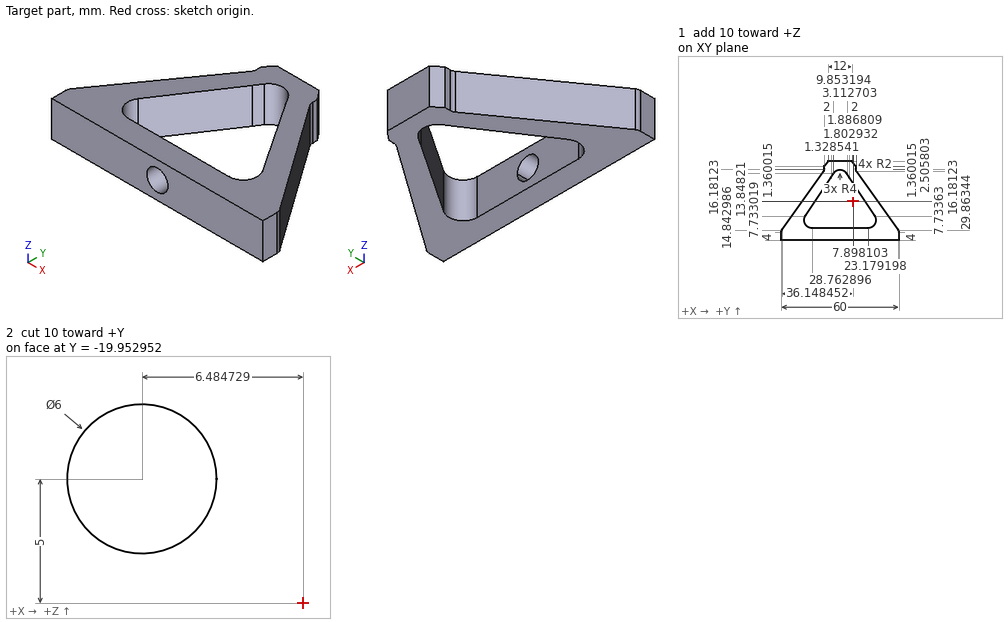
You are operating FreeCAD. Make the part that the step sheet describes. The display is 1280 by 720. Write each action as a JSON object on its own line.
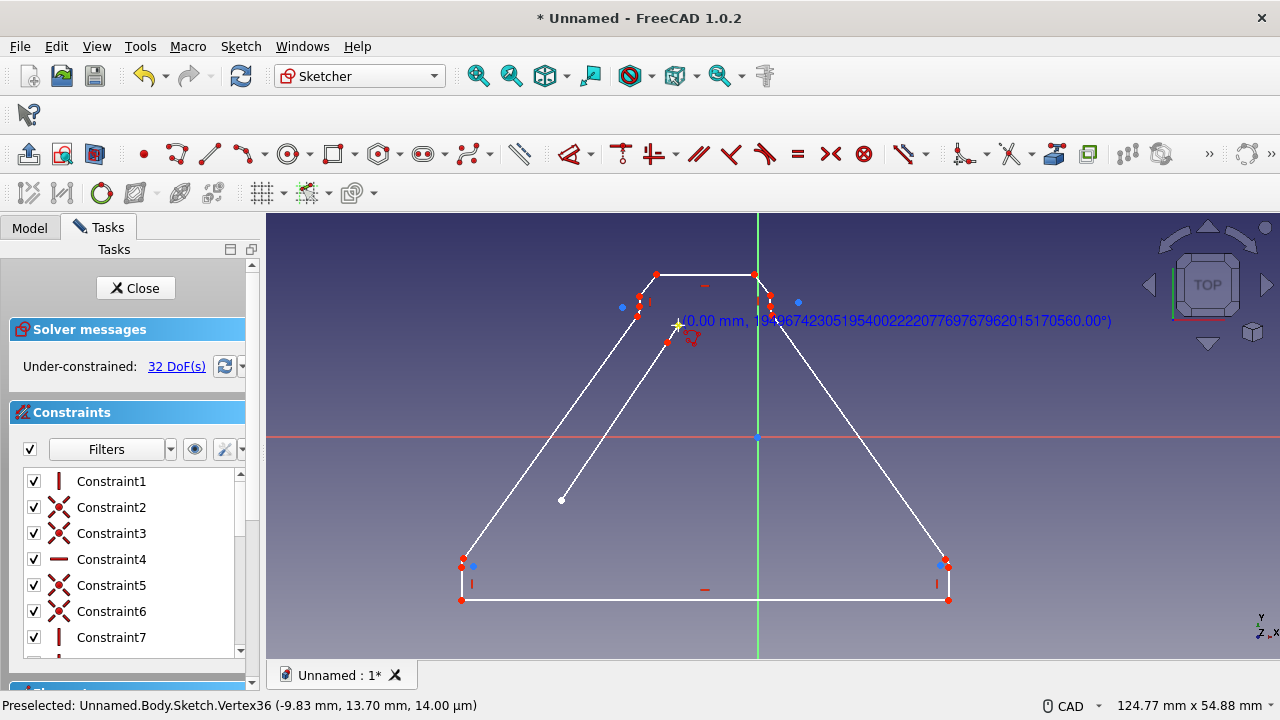
{"action": "left_click", "coordinate": [733, 325]}
{"action": "left_click", "coordinate": [743, 341]}
{"action": "left_click", "coordinate": [849, 500]}
{"action": "right_click", "coordinate": [849, 500]}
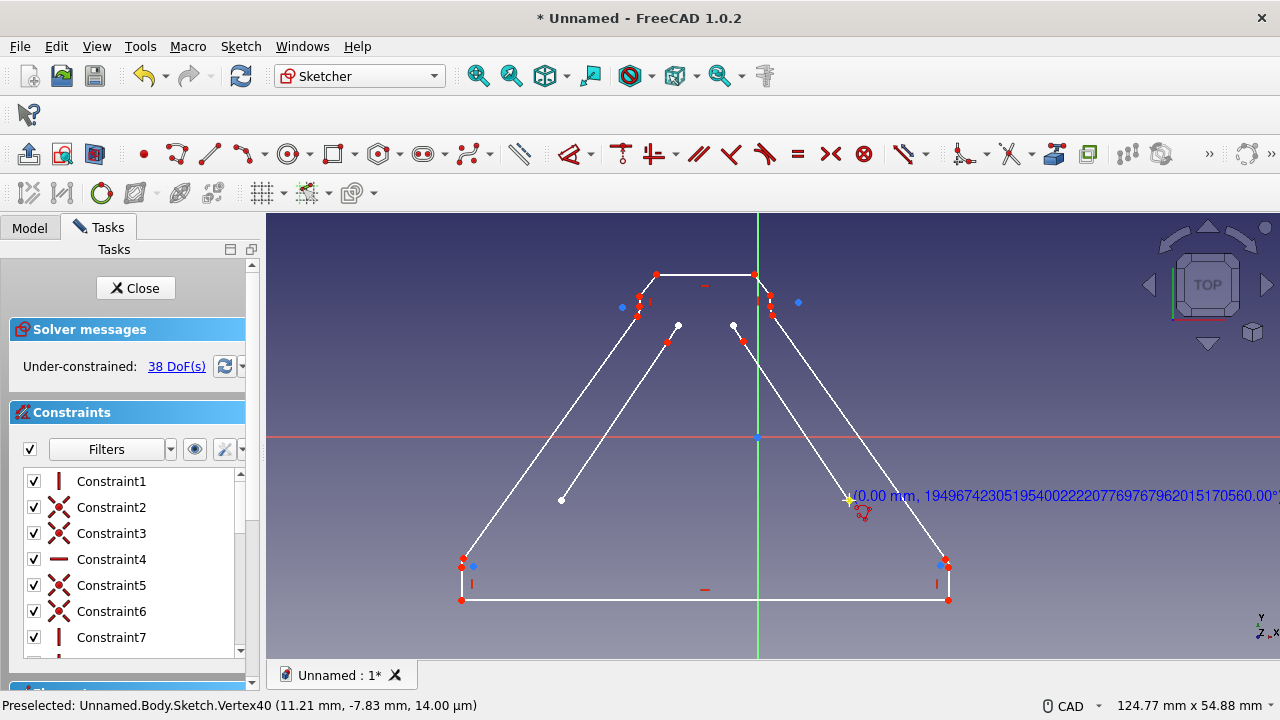
{"action": "left_click", "coordinate": [210, 154]}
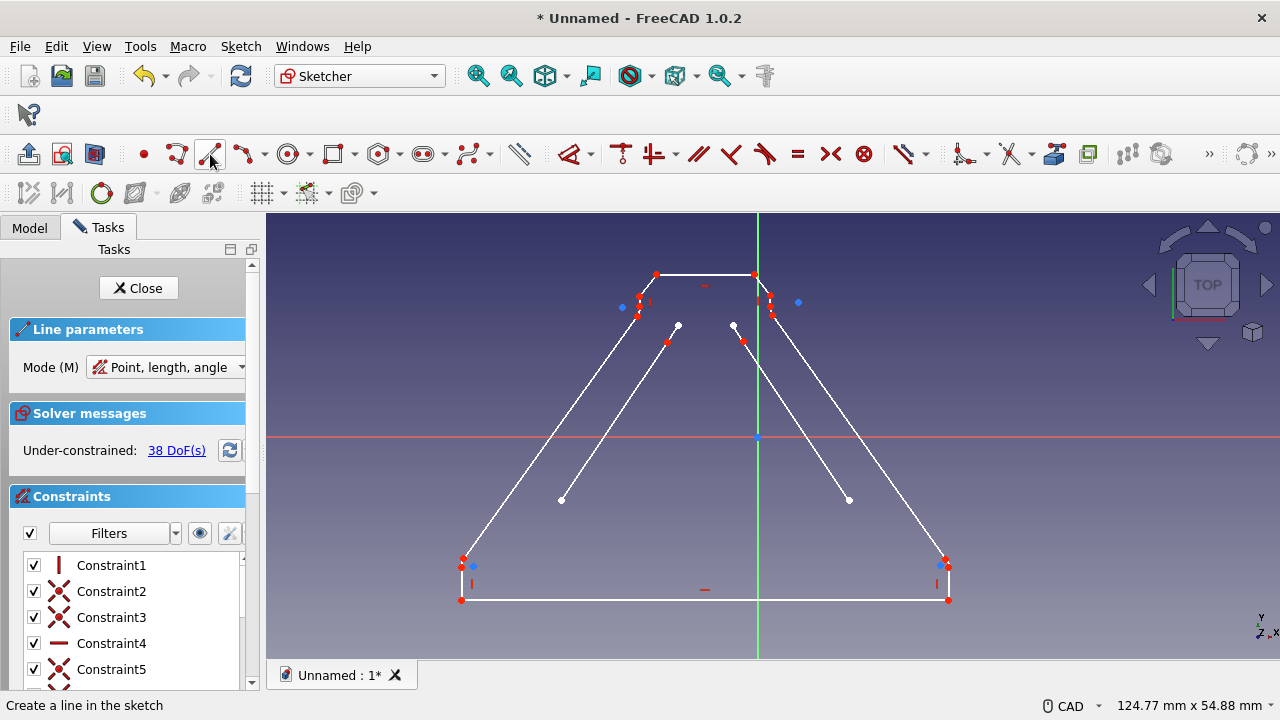
{"action": "left_click", "coordinate": [822, 551]}
{"action": "left_click", "coordinate": [588, 551]}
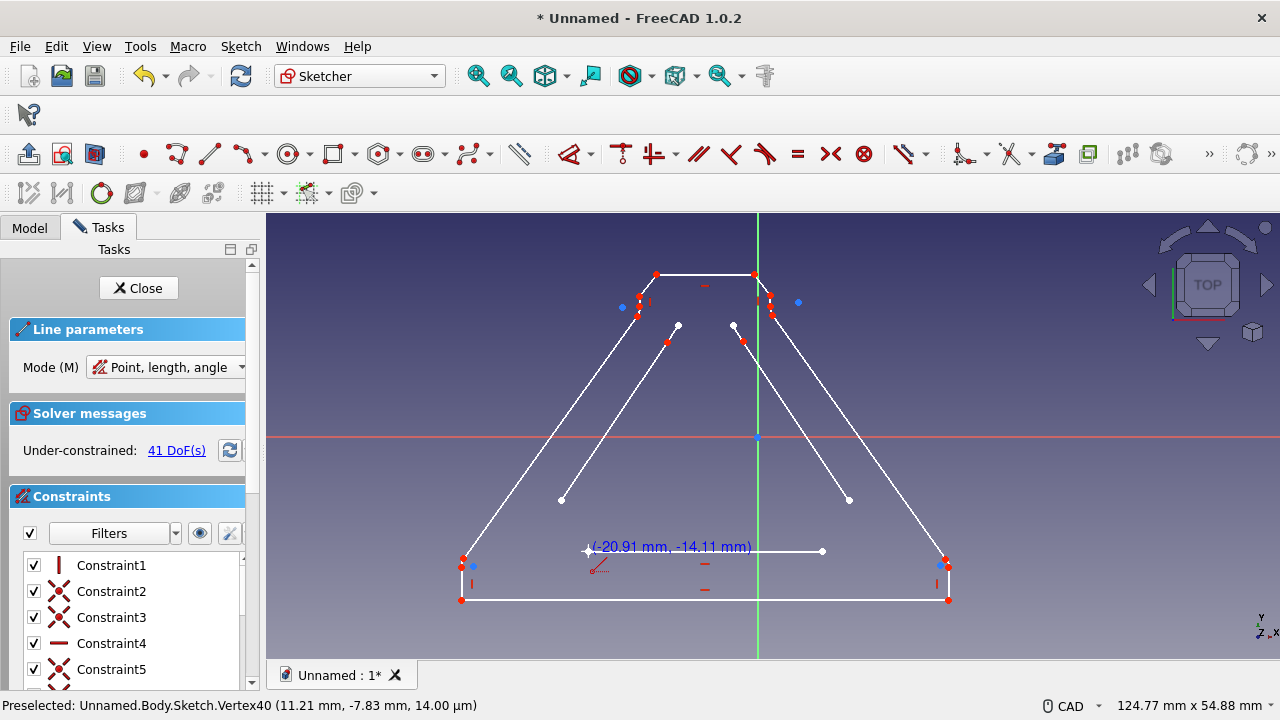
{"action": "left_click", "coordinate": [242, 154]}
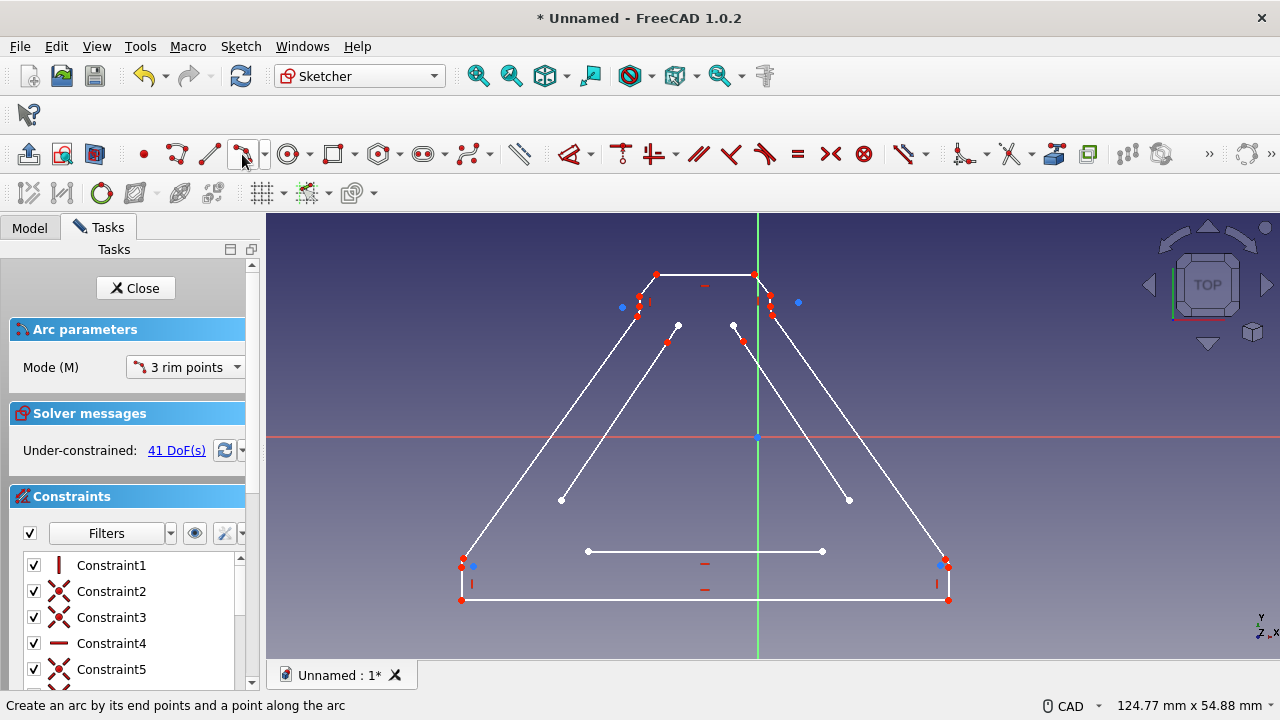
{"action": "scroll", "coordinate": [678, 325], "scroll_direction": "up", "scroll_amount": 3}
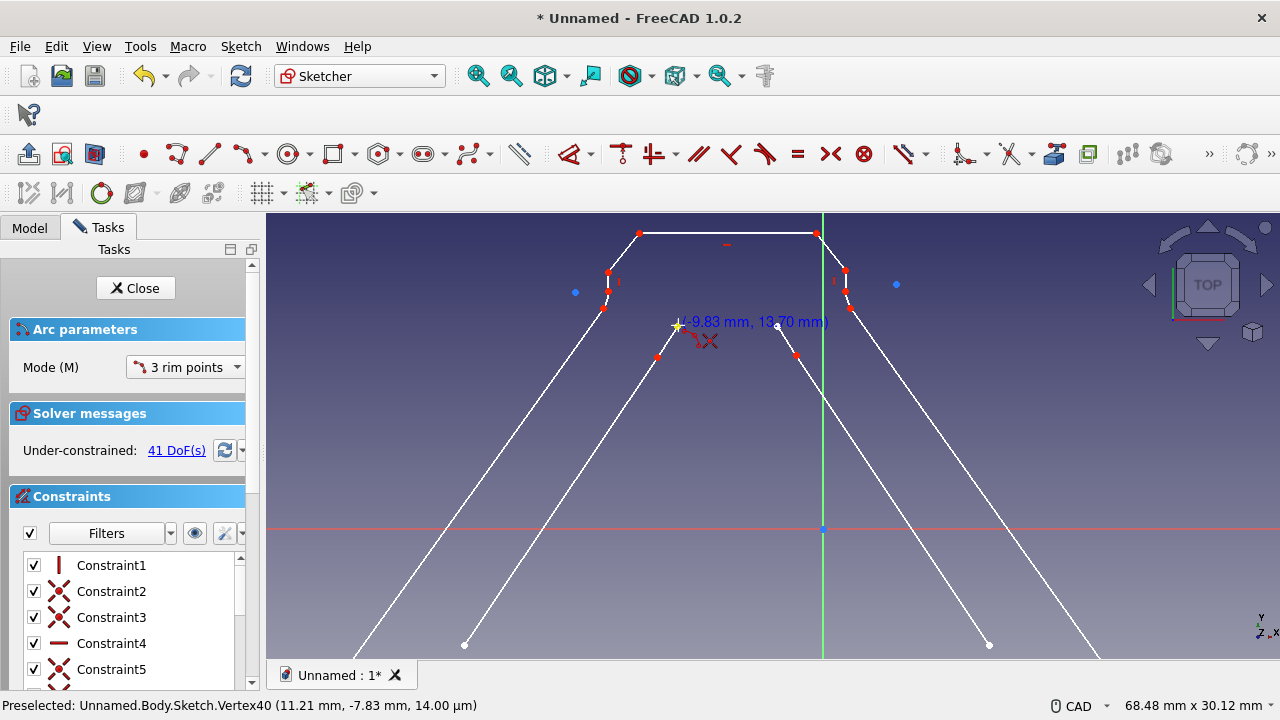
{"action": "left_click", "coordinate": [678, 327]}
{"action": "left_click", "coordinate": [778, 327]}
{"action": "left_click", "coordinate": [727, 297]}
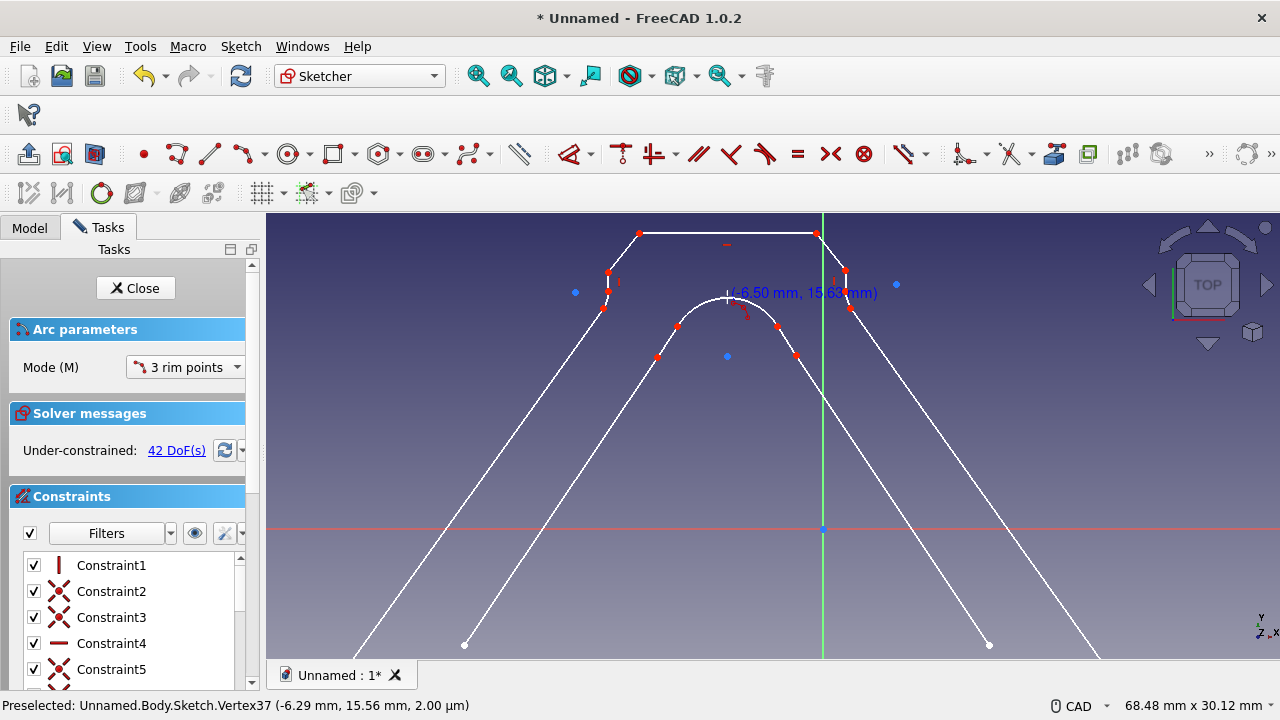
{"action": "scroll", "coordinate": [686, 360], "scroll_direction": "down", "scroll_amount": 4}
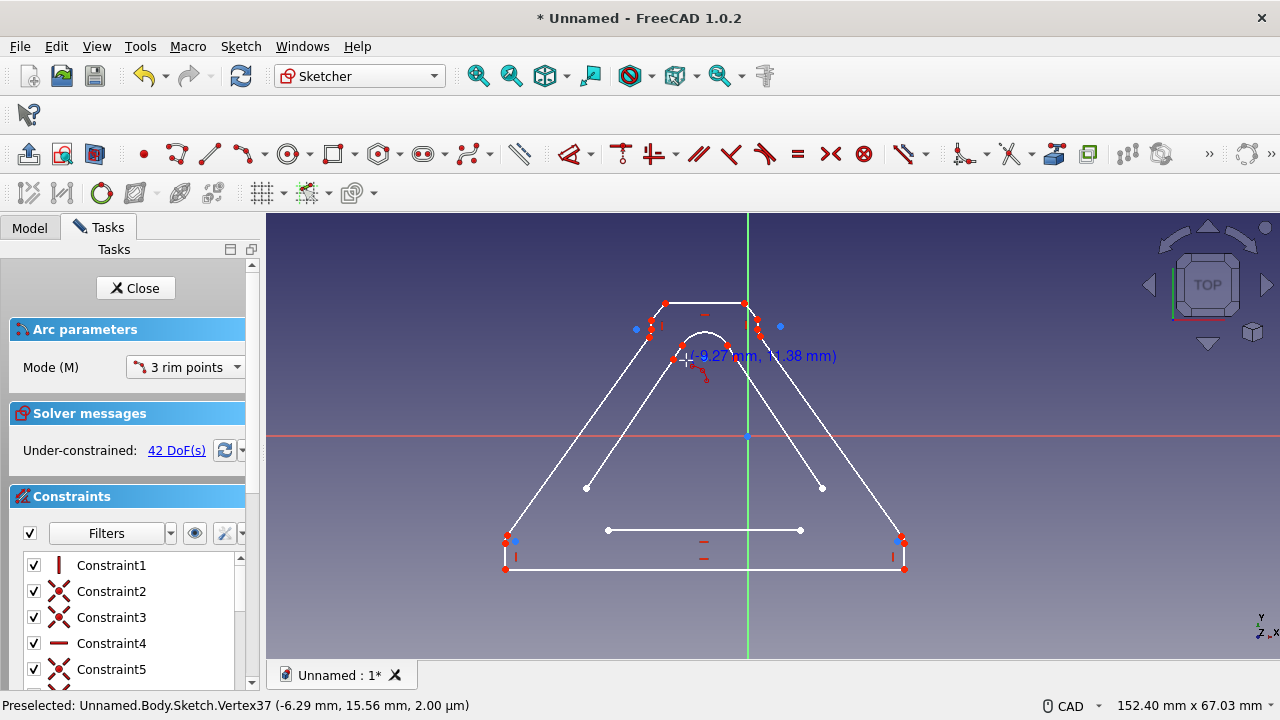
{"action": "left_click", "coordinate": [822, 488]}
{"action": "left_click", "coordinate": [800, 530]}
{"action": "left_click", "coordinate": [824, 515]}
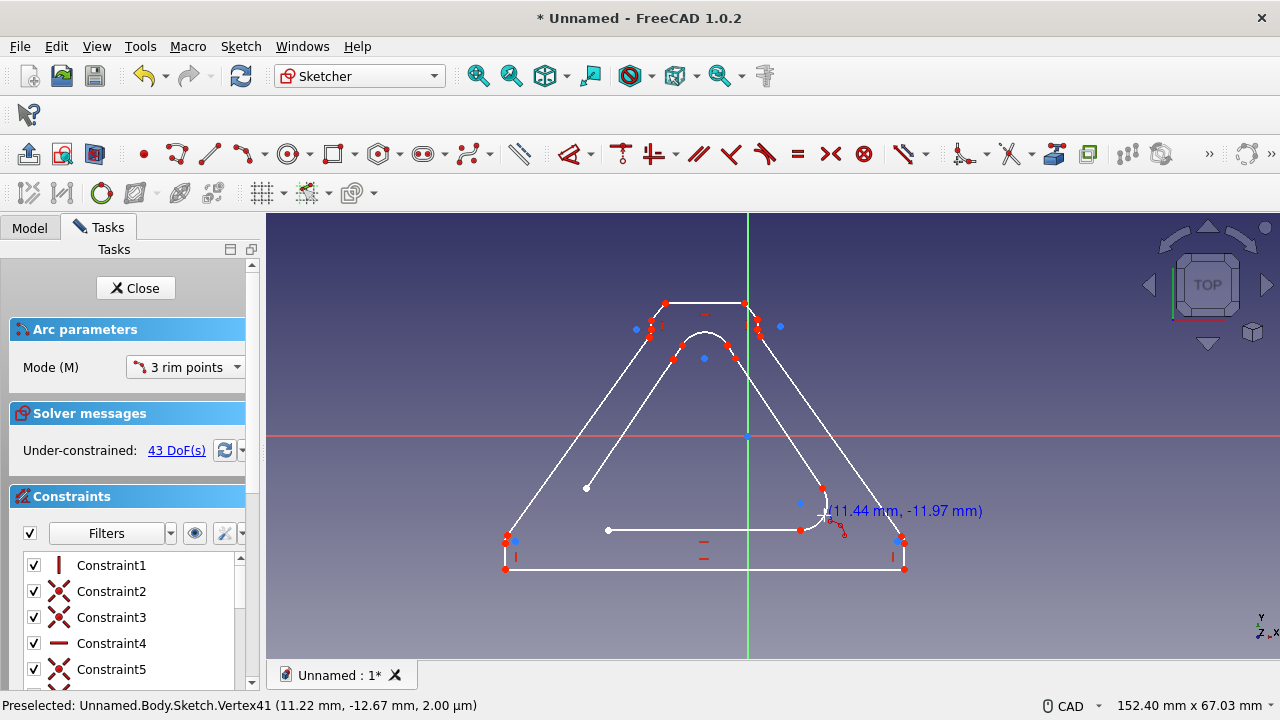
{"action": "left_click", "coordinate": [609, 530]}
{"action": "left_click", "coordinate": [587, 488]}
{"action": "left_click", "coordinate": [586, 515]}
{"action": "key", "text": "Escape"}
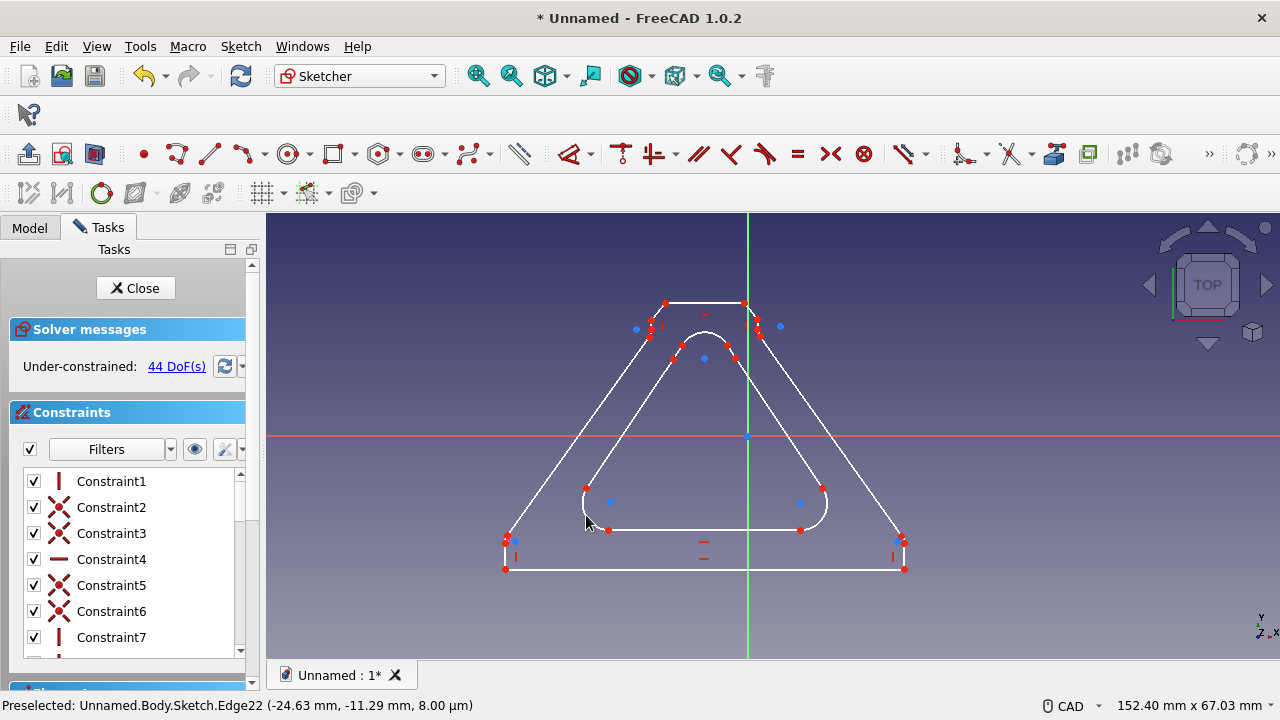
{"action": "left_click", "coordinate": [859, 476]}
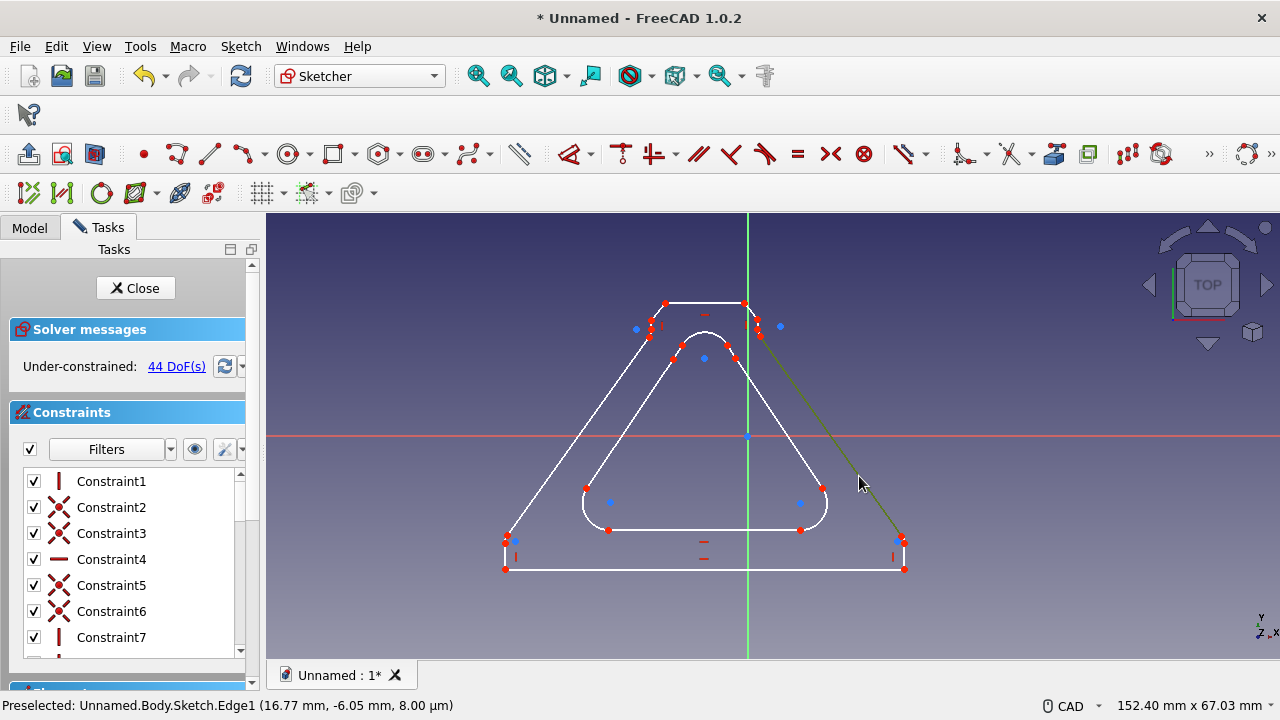
{"action": "scroll", "coordinate": [759, 333], "scroll_direction": "up", "scroll_amount": 7}